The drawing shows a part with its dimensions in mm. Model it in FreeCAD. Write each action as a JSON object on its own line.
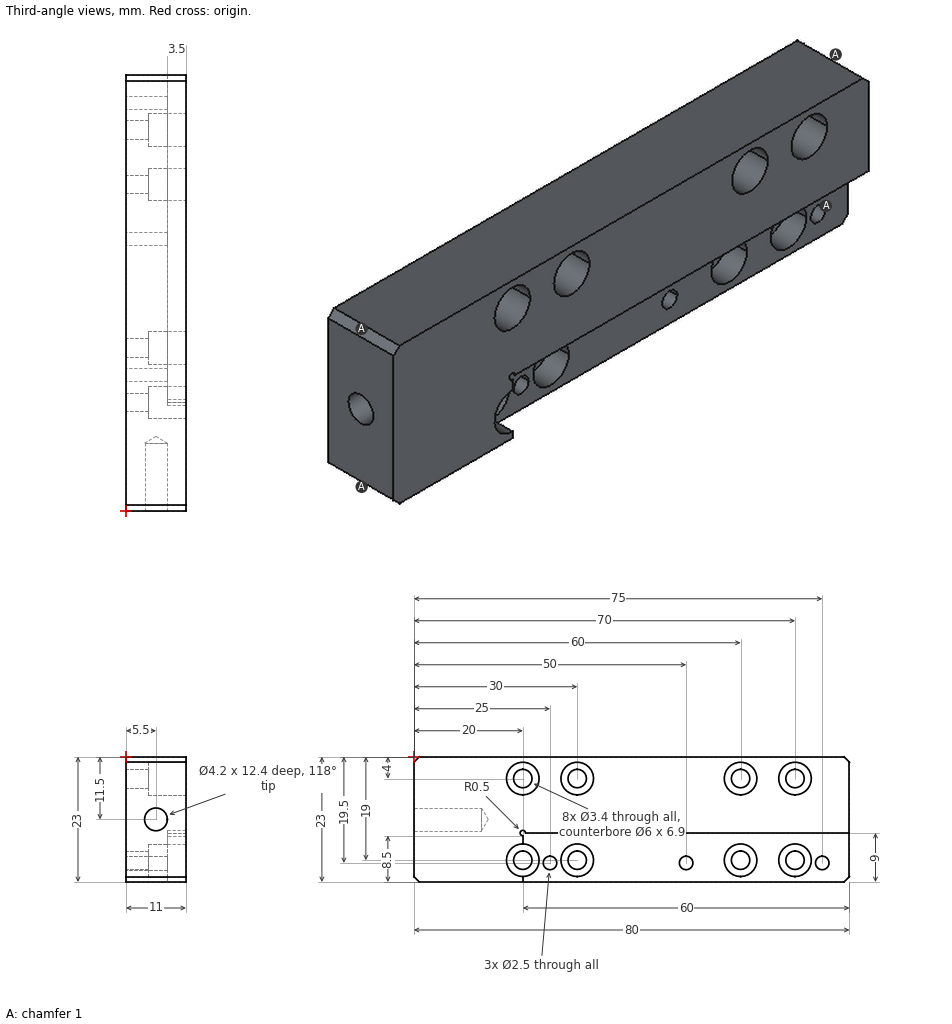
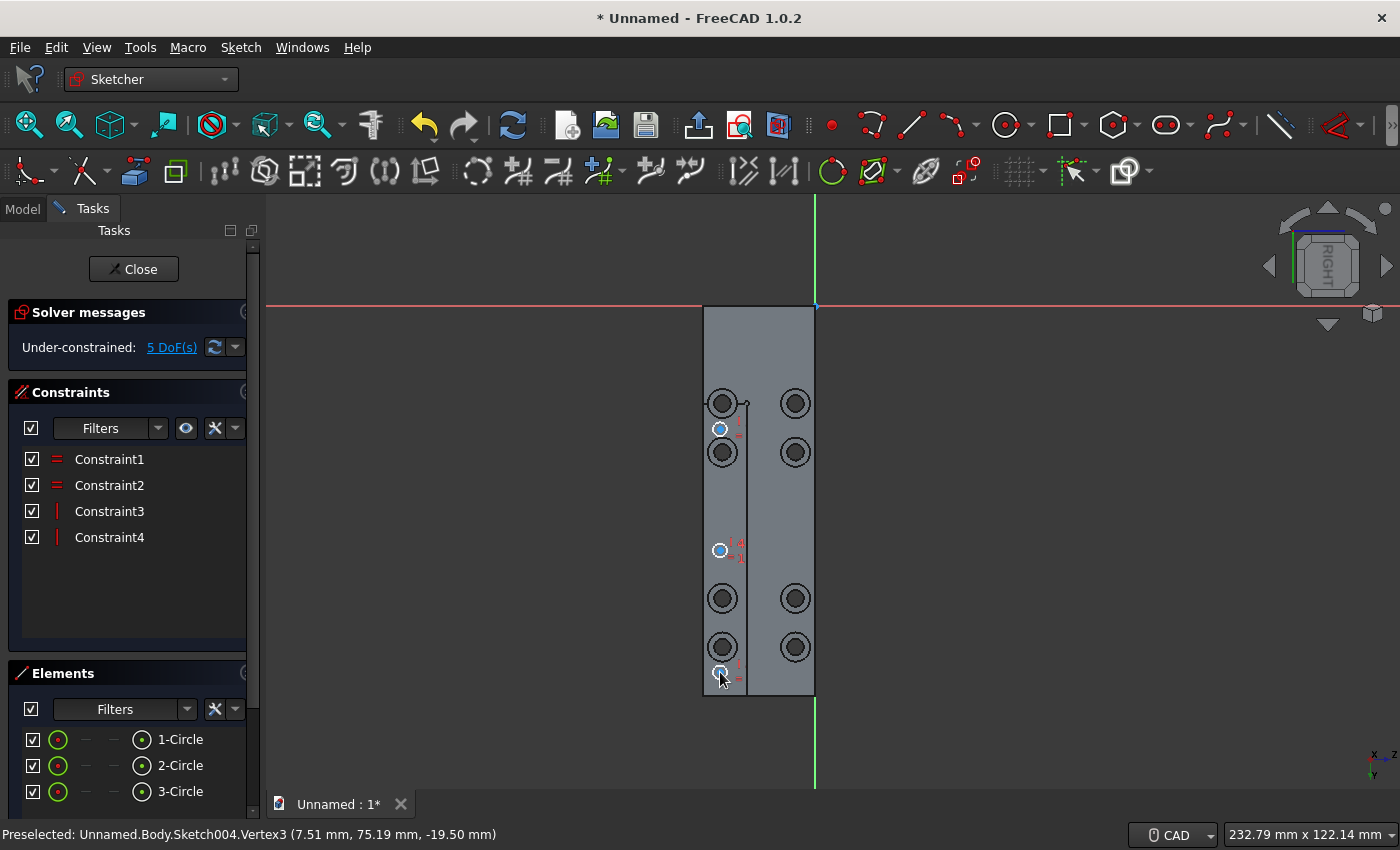
{"action": "left_click", "coordinate": [1336, 126]}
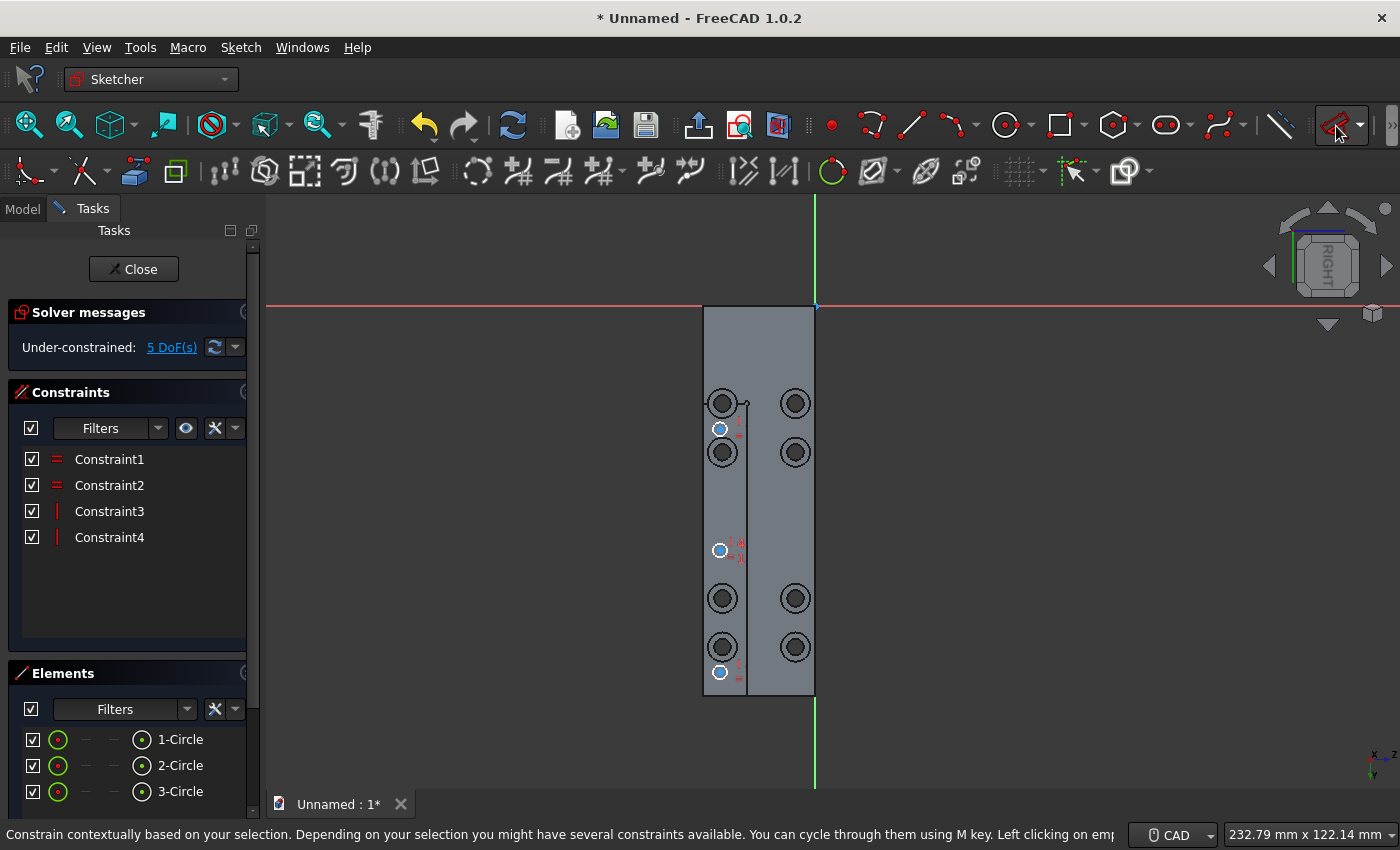
{"action": "scroll", "coordinate": [720, 422], "scroll_direction": "up", "scroll_amount": 6}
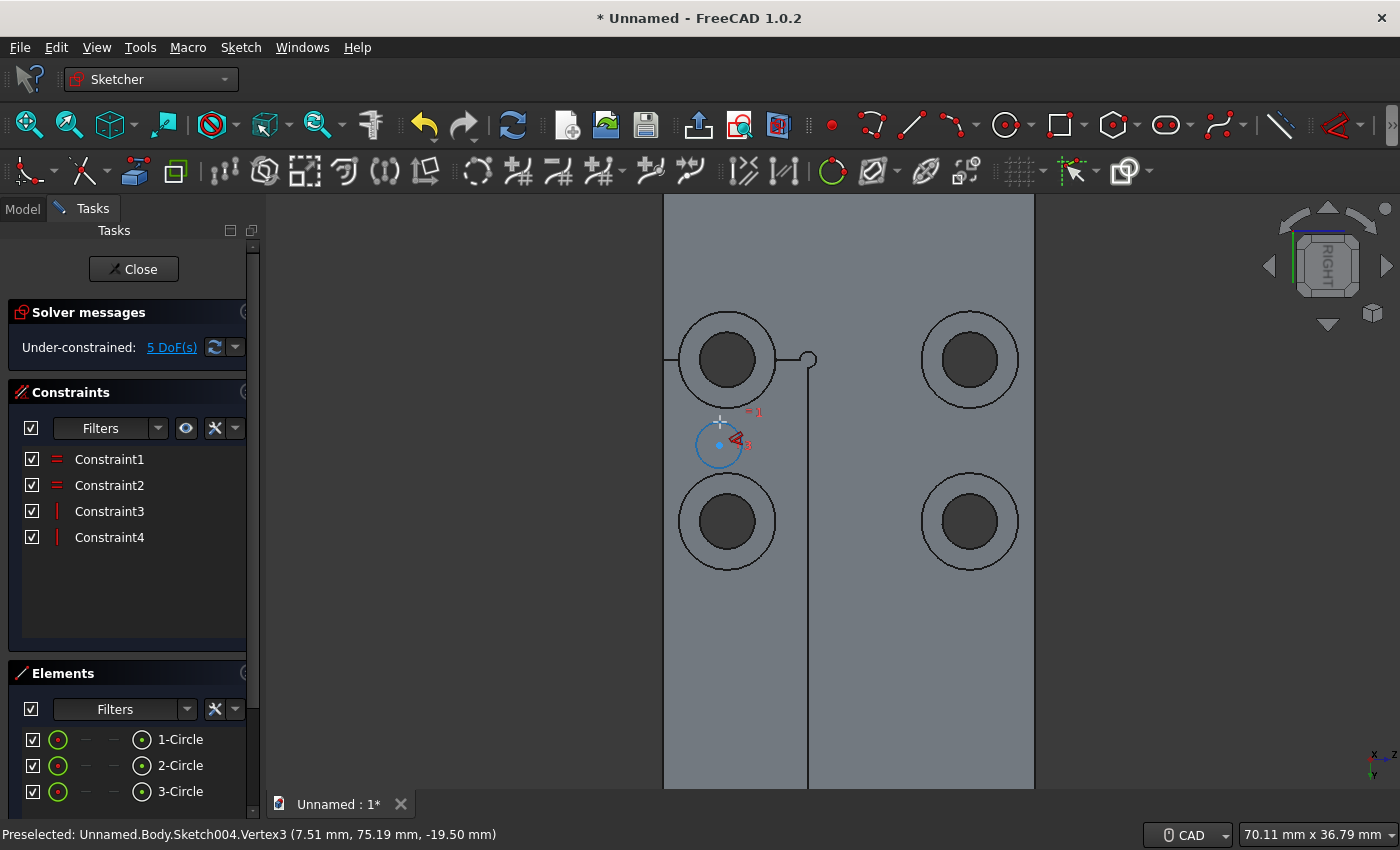
{"action": "left_click", "coordinate": [720, 422]}
{"action": "left_click", "coordinate": [721, 390]}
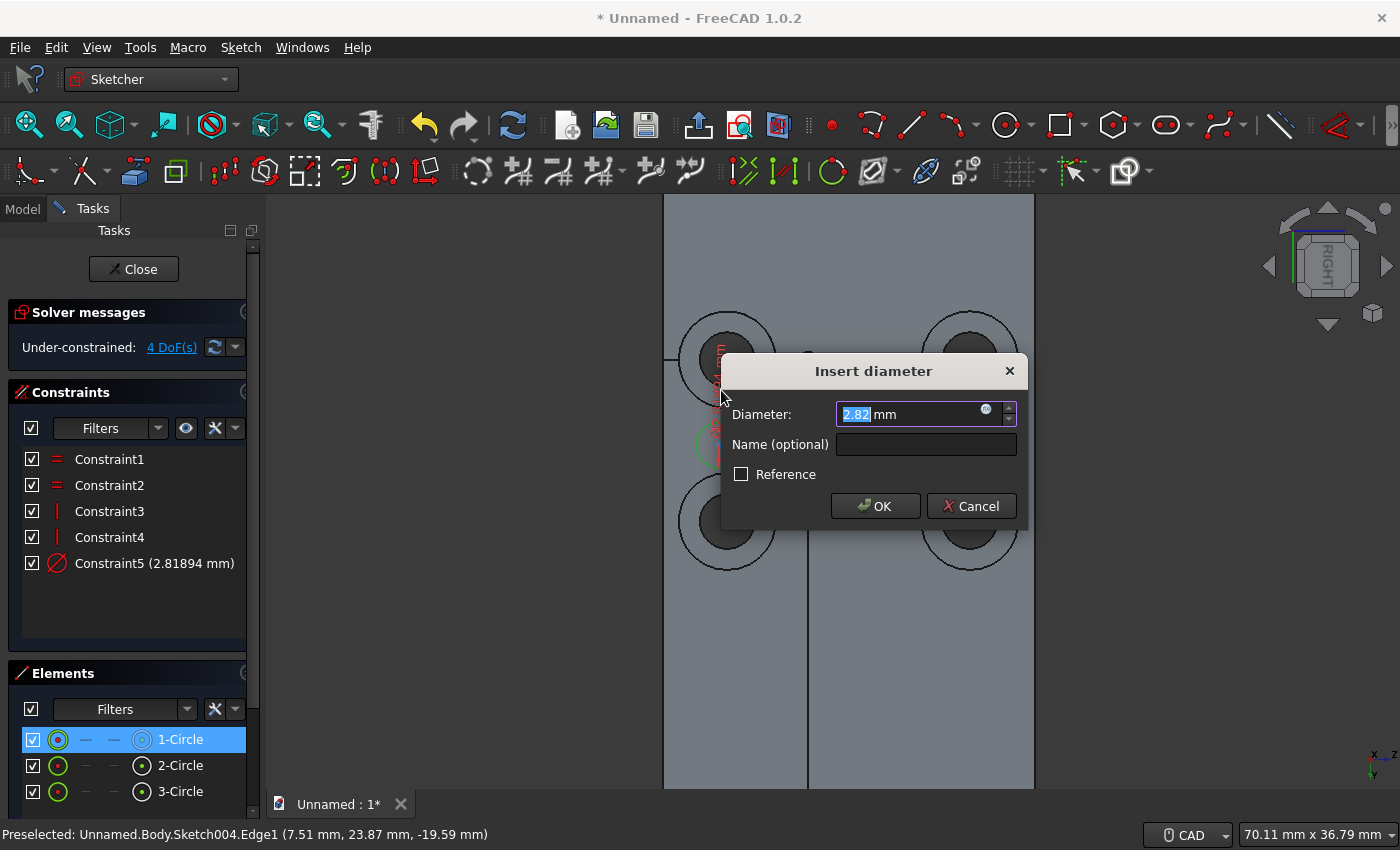
{"action": "type", "text": "2.5"}
{"action": "key", "text": "Return"}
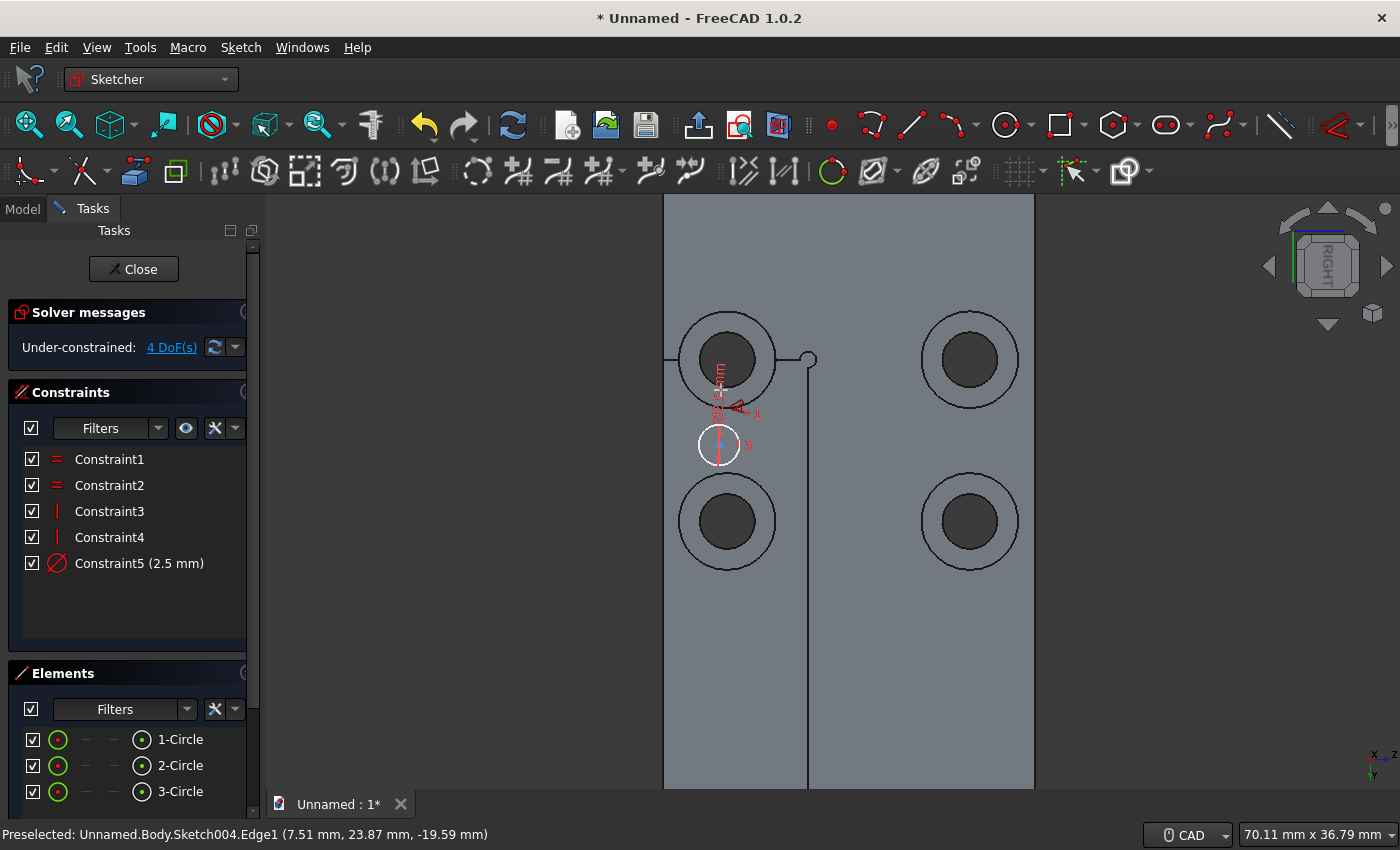
{"action": "scroll", "coordinate": [720, 422], "scroll_direction": "down", "scroll_amount": 6}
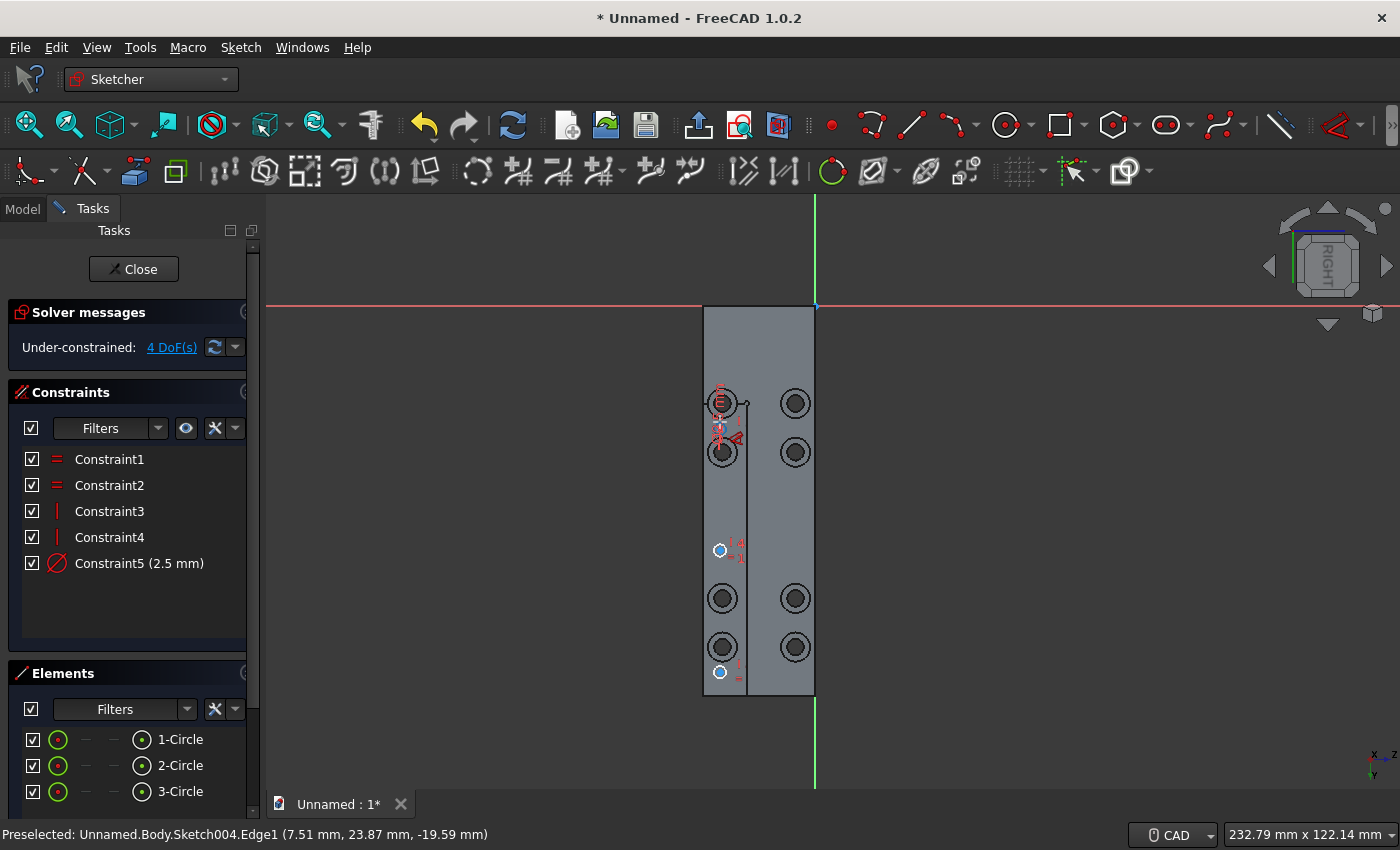
{"action": "left_click", "coordinate": [720, 429]}
{"action": "left_click", "coordinate": [849, 368]}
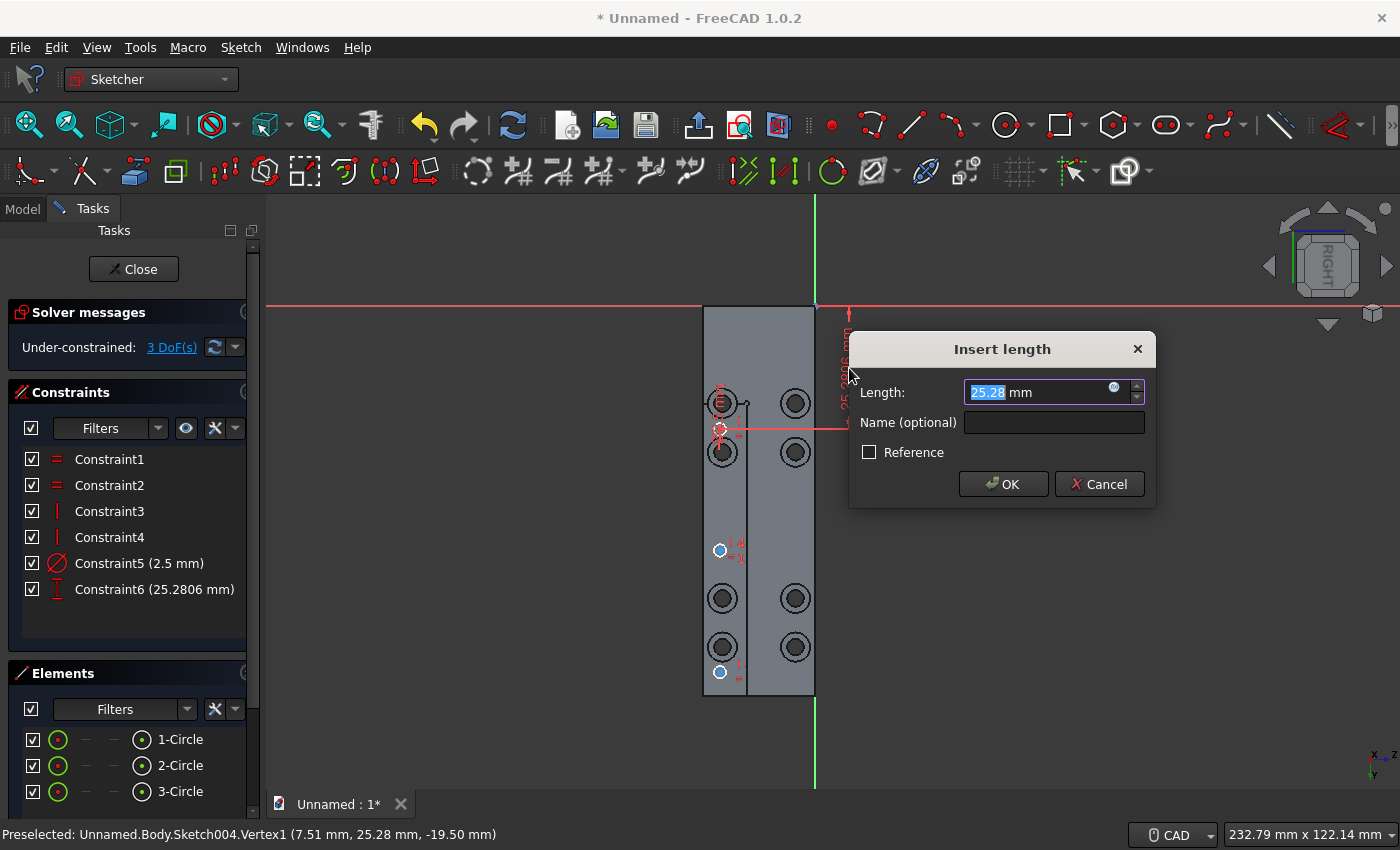
{"action": "type", "text": "25"}
{"action": "key", "text": "Return"}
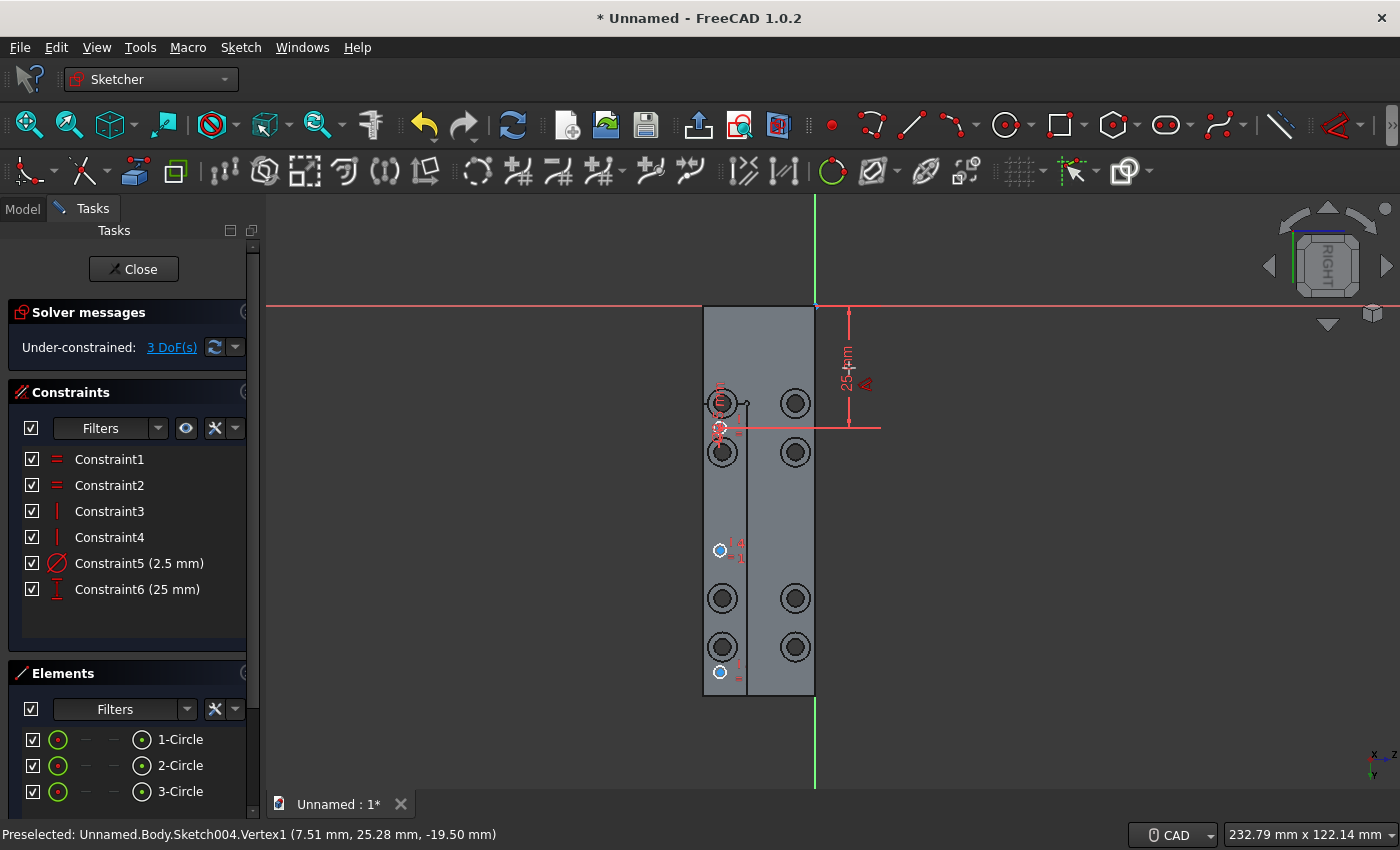
{"action": "left_click", "coordinate": [720, 550]}
{"action": "left_click", "coordinate": [849, 428]}